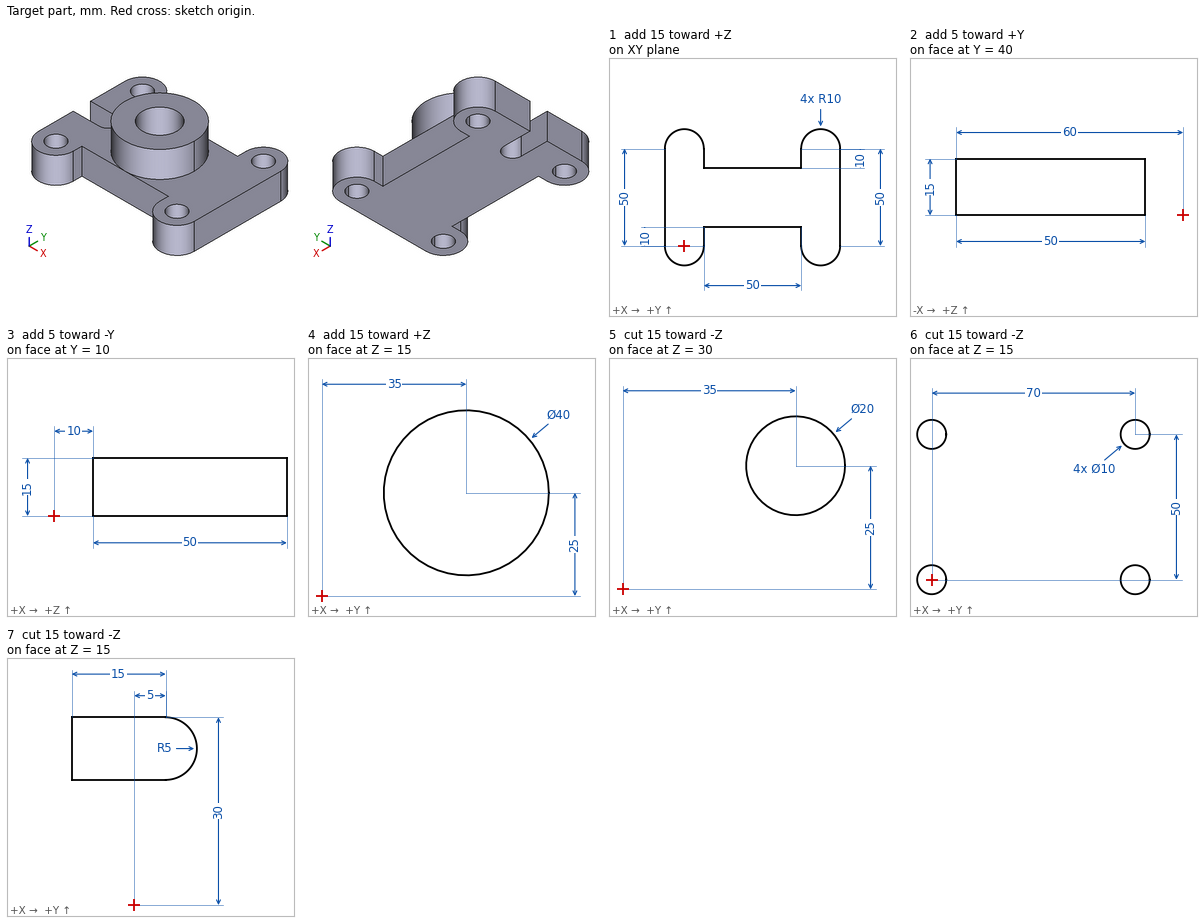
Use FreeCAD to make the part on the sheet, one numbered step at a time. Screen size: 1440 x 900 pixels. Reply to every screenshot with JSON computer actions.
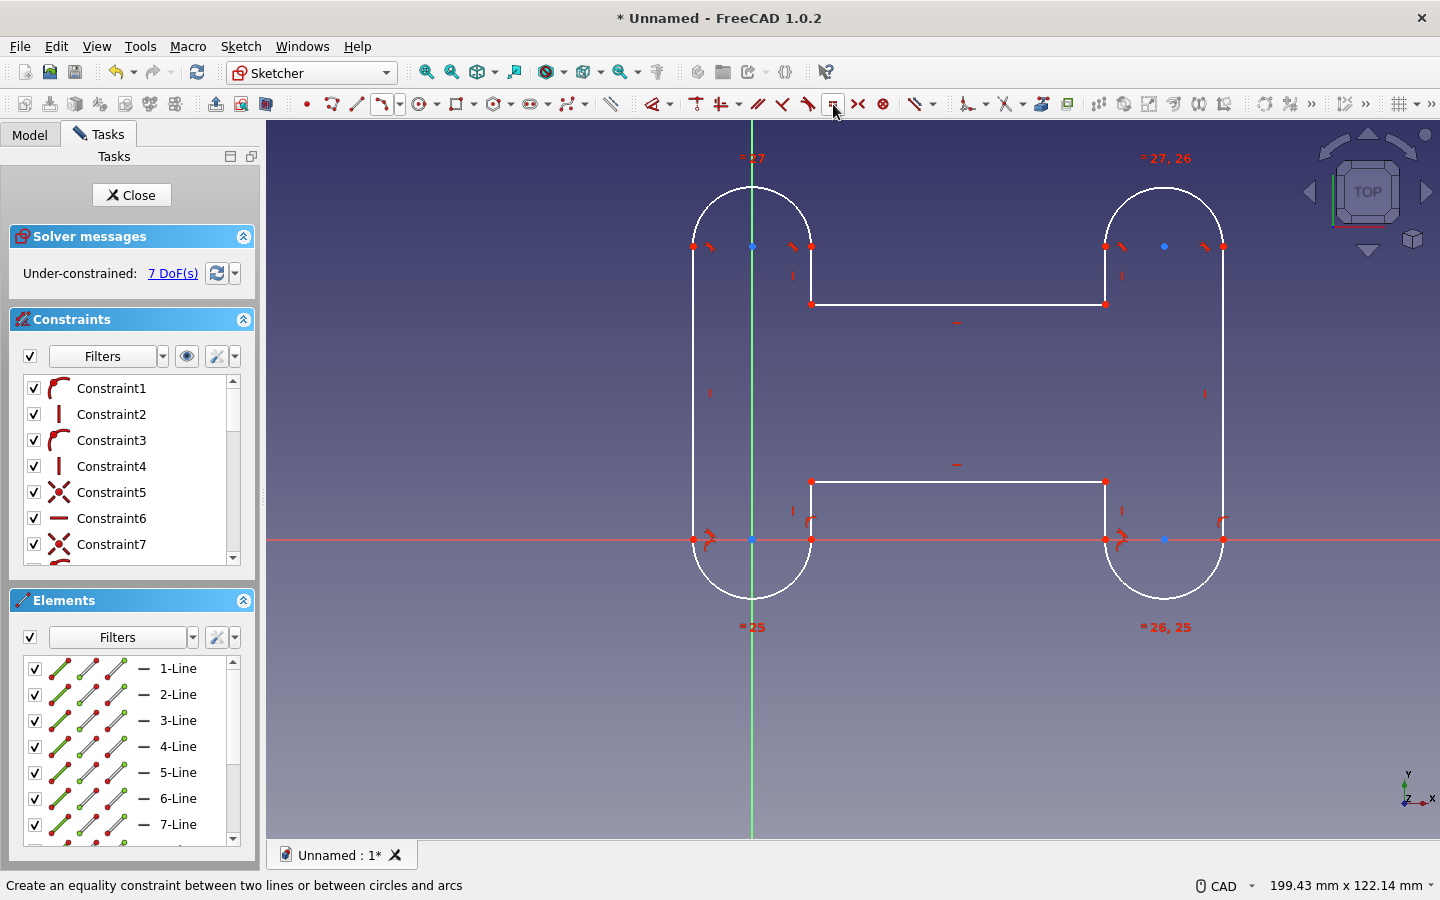
{"action": "left_click", "coordinate": [752, 540]}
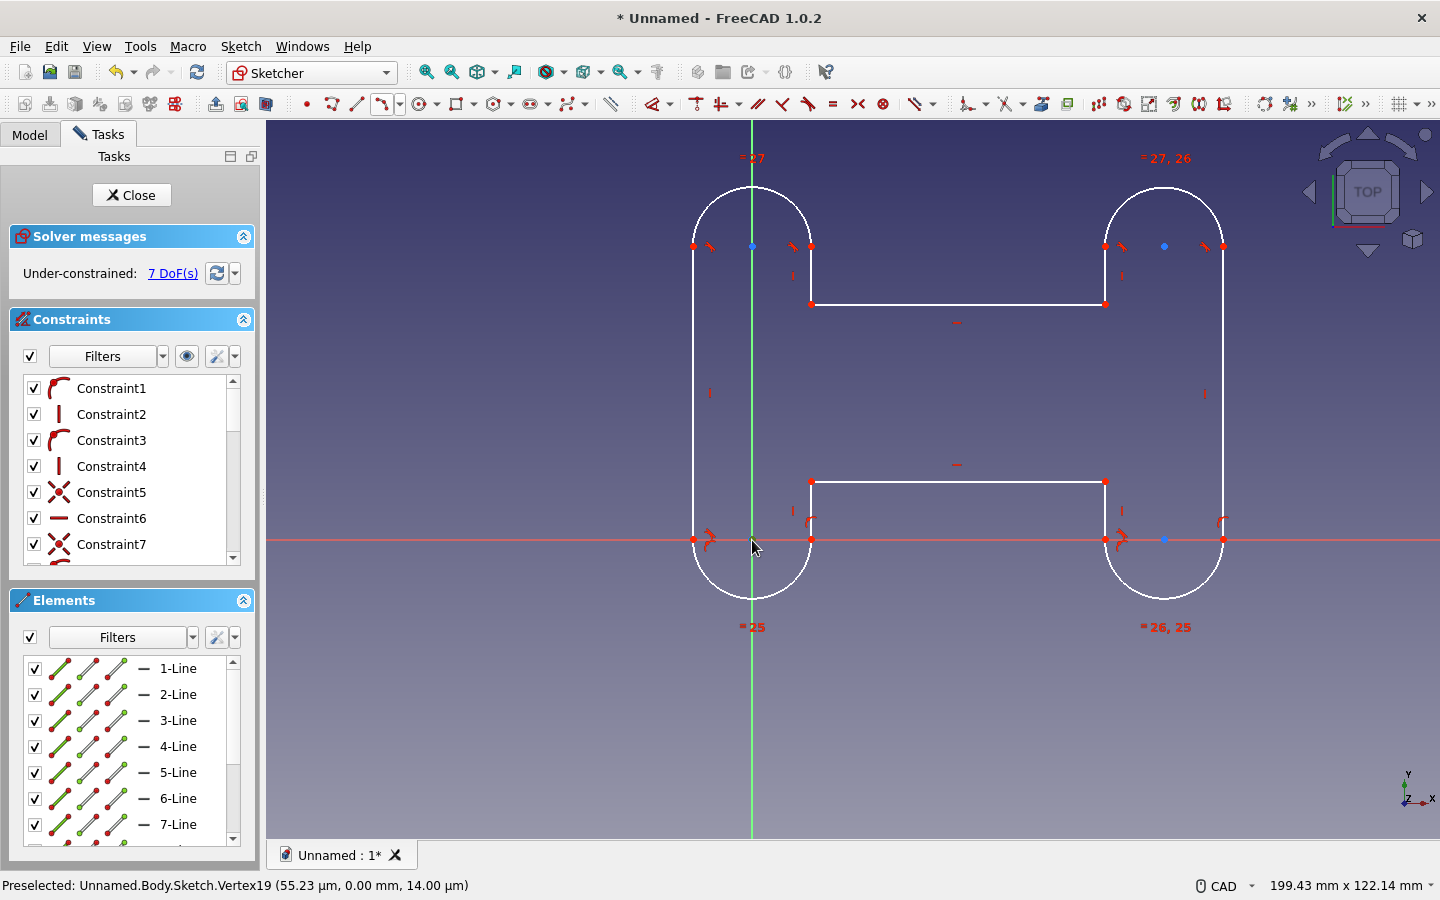
{"action": "left_click", "coordinate": [752, 764]}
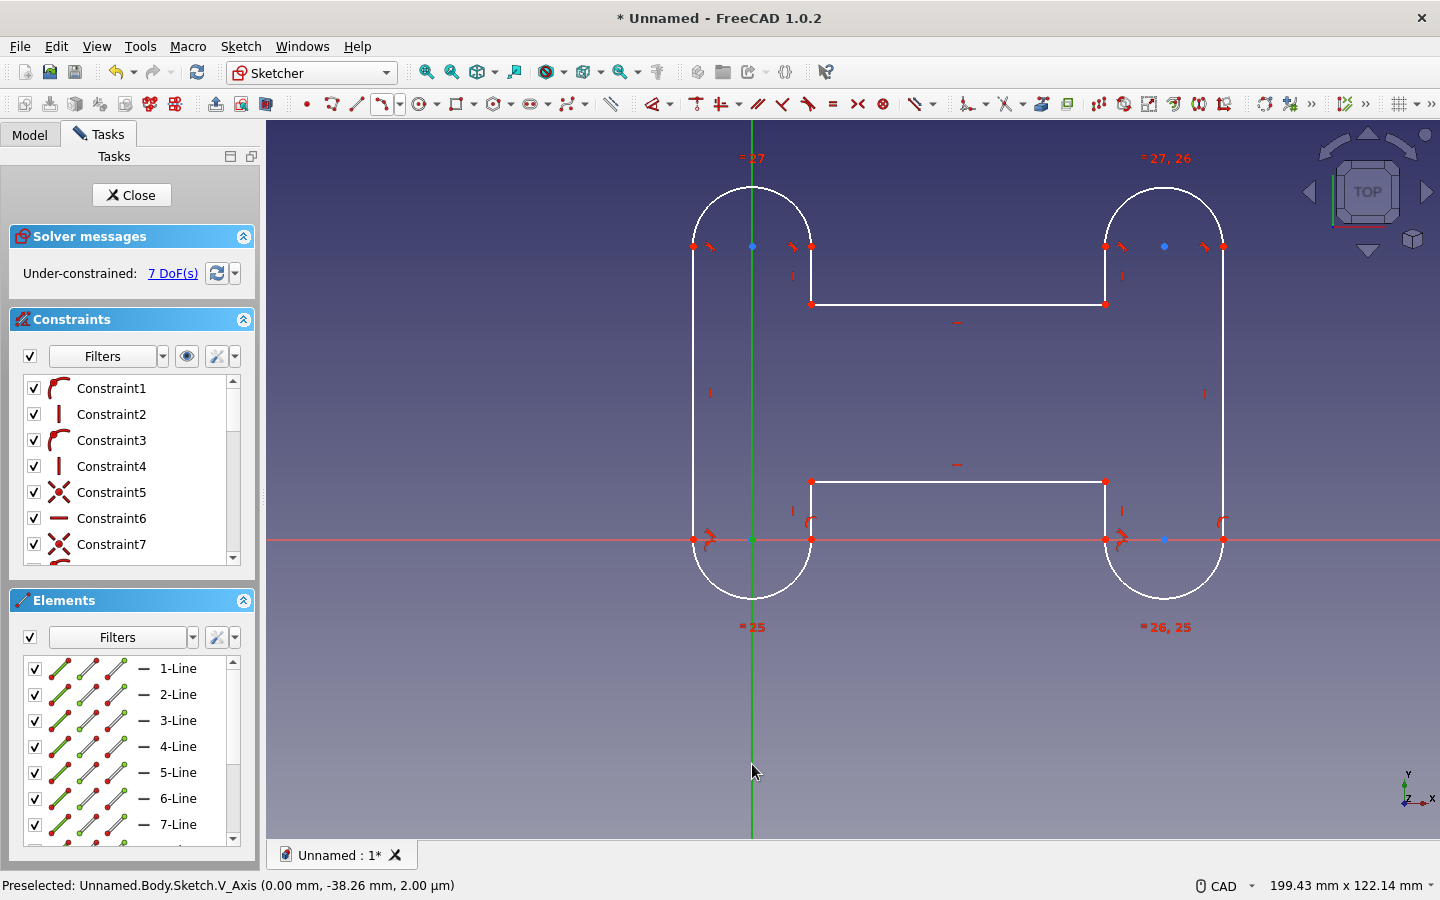
{"action": "key", "text": "c"}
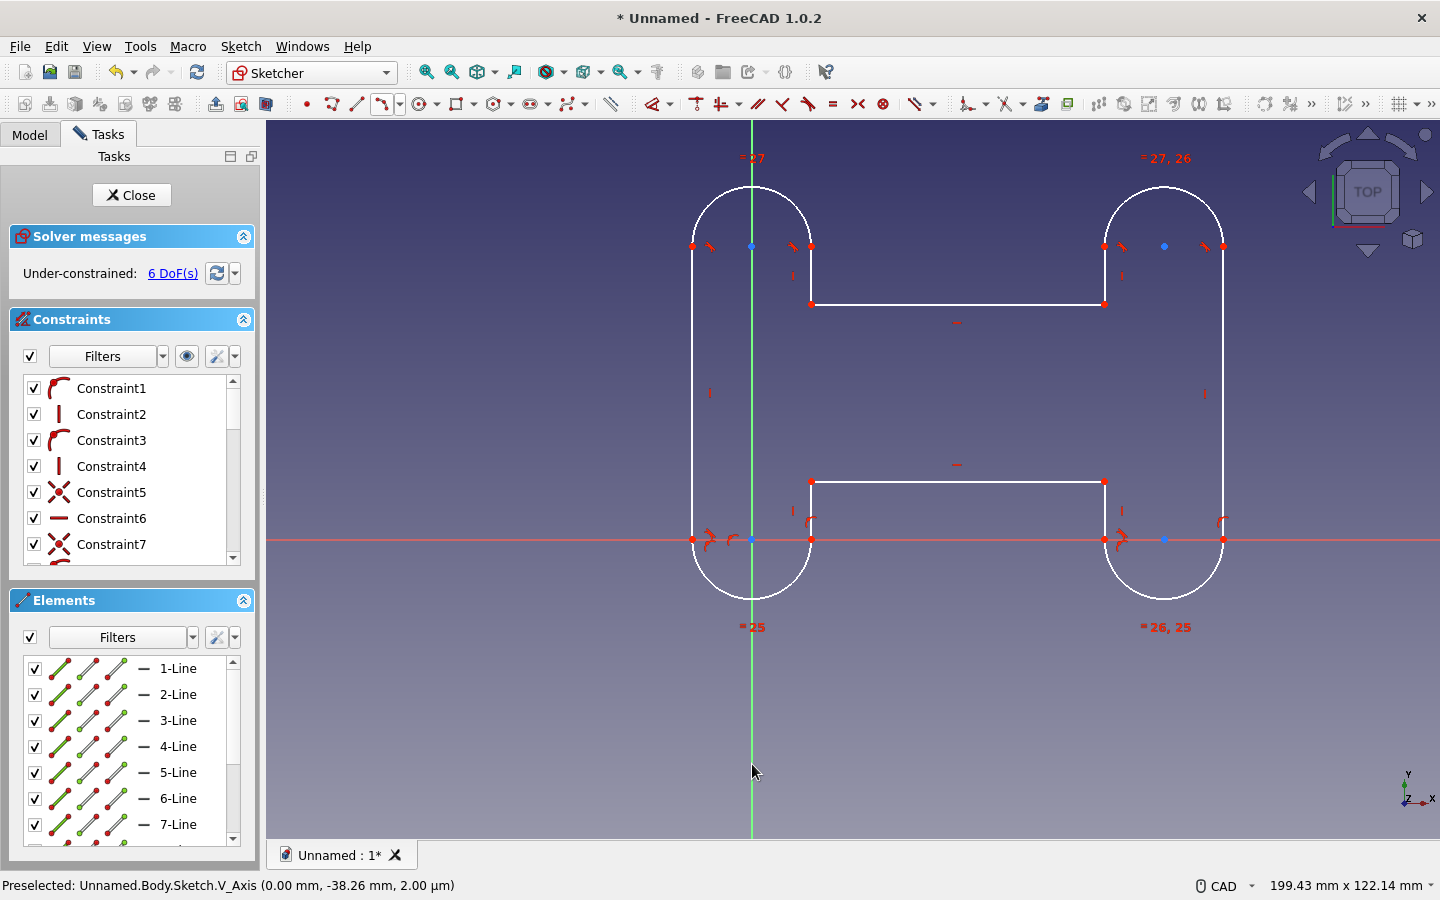
{"action": "left_click", "coordinate": [717, 588]}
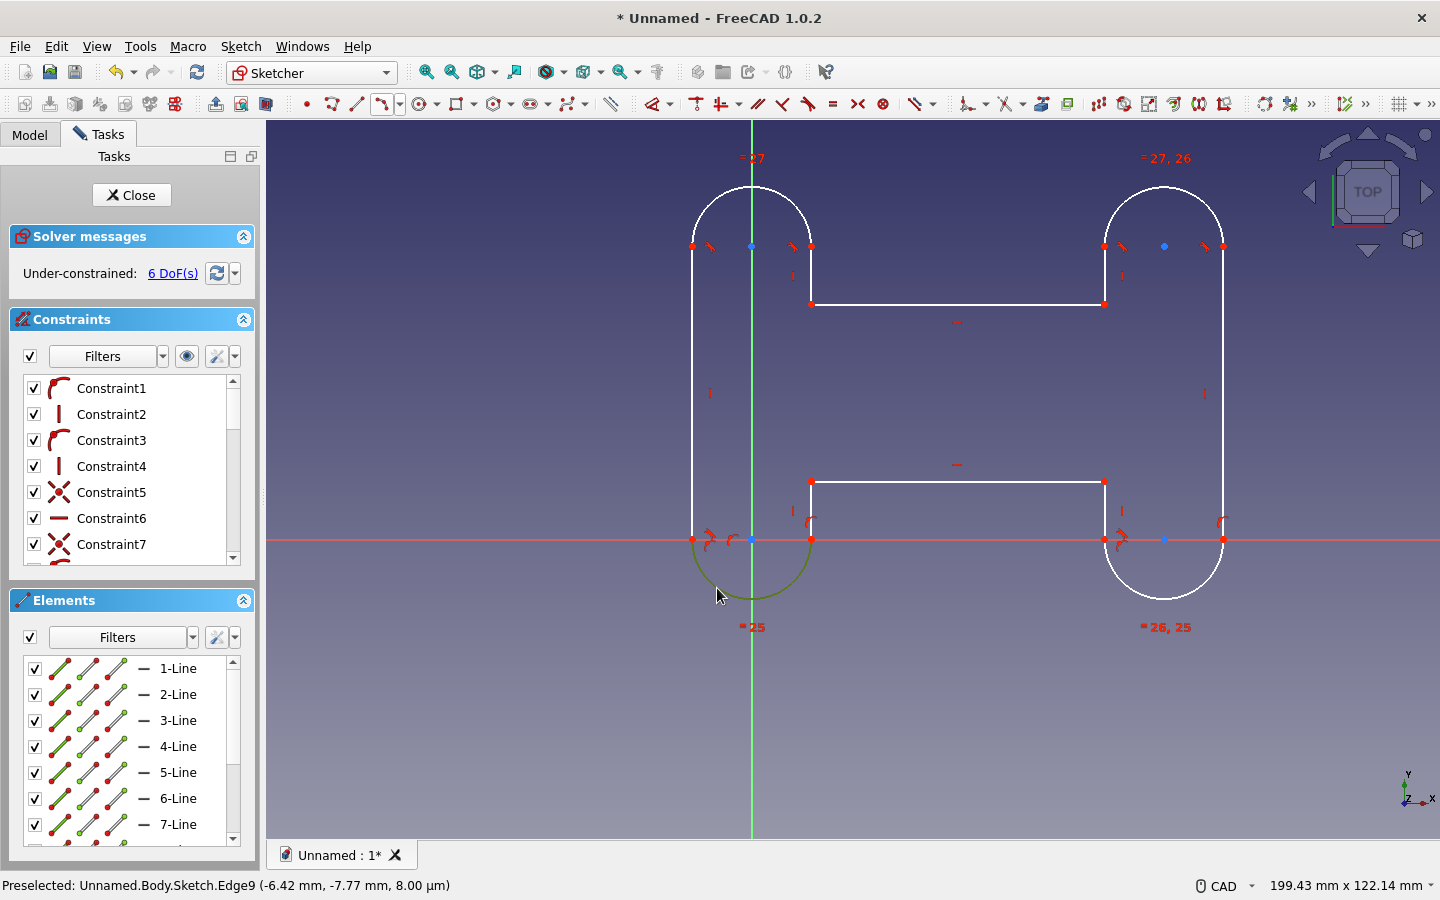
{"action": "key", "text": "k r"}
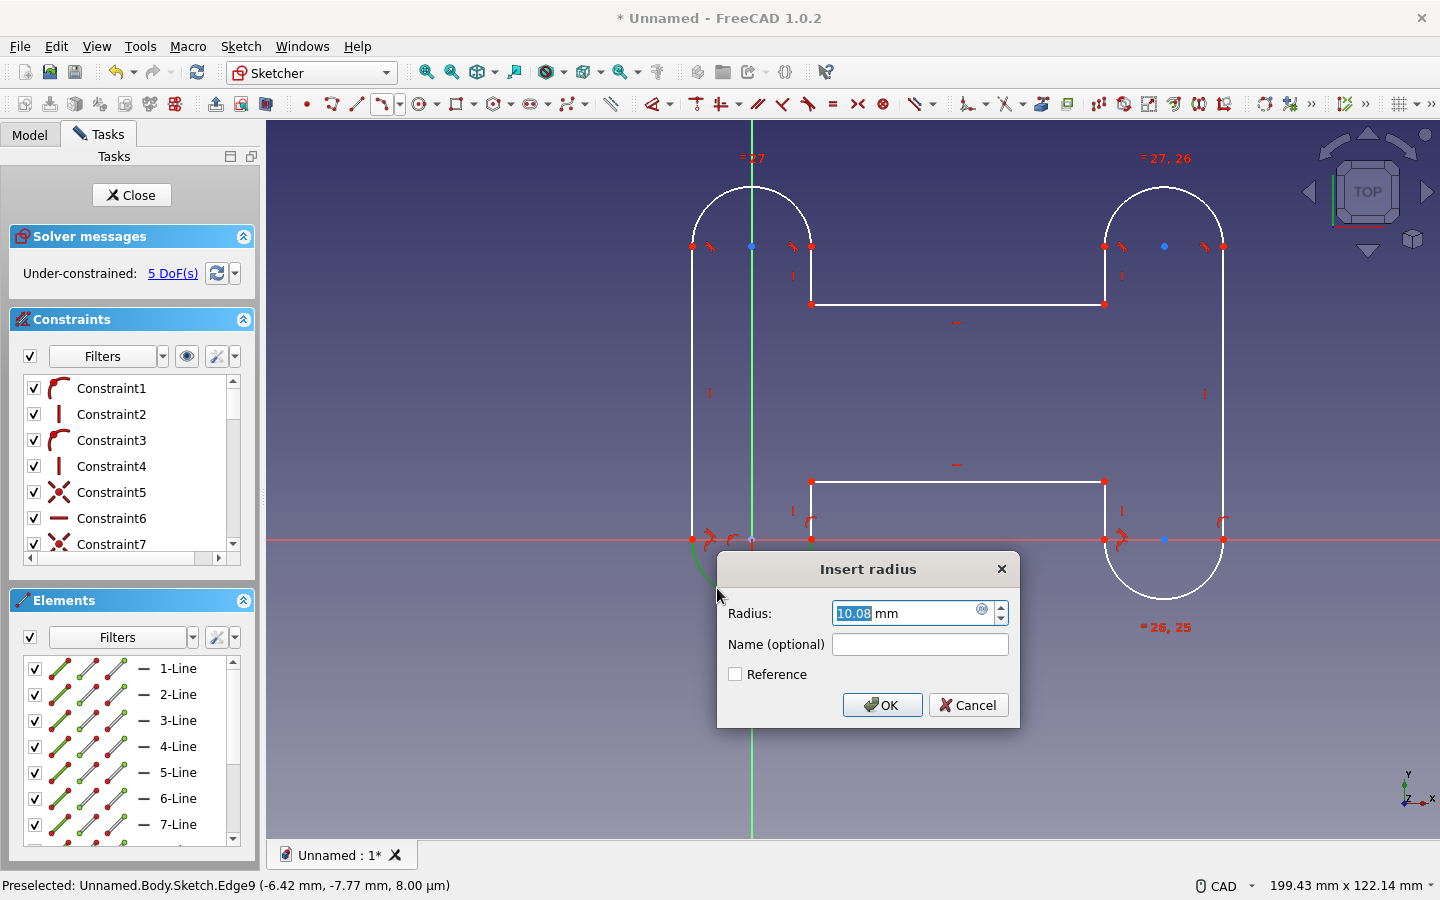
{"action": "type", "text": "10"}
{"action": "key", "text": "Return"}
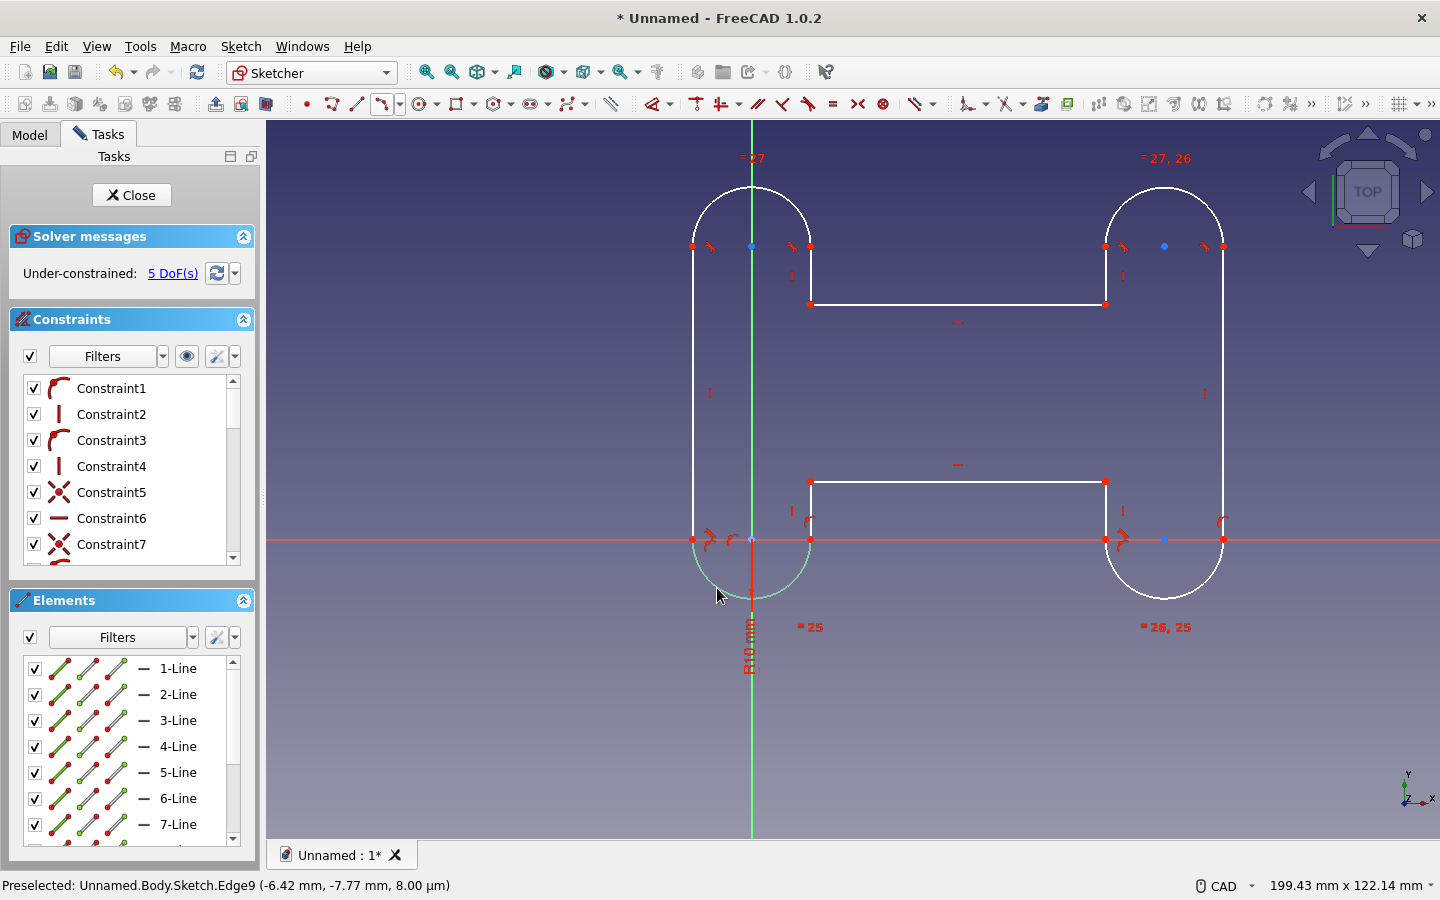
{"action": "left_click", "coordinate": [693, 334]}